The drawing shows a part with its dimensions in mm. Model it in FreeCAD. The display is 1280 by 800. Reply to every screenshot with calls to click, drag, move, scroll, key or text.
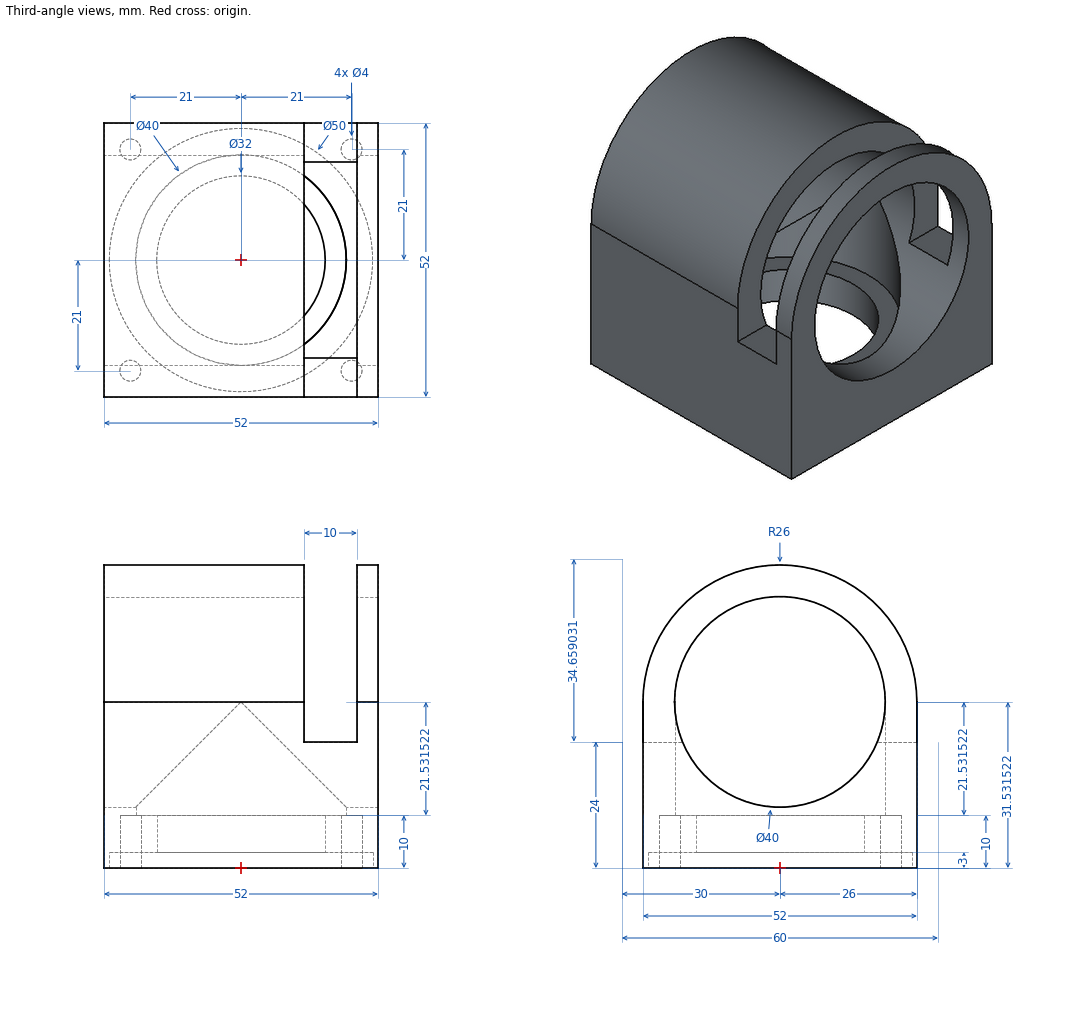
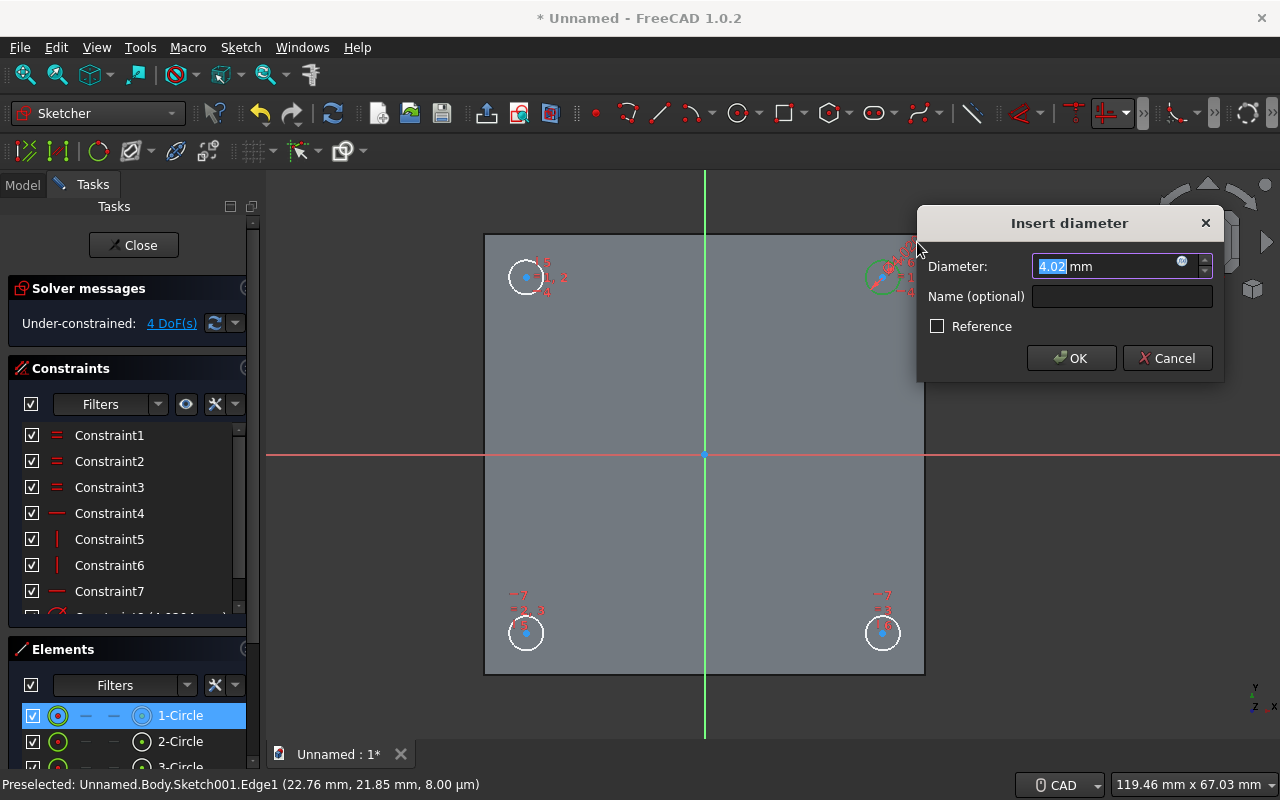
text(4)
key(Return)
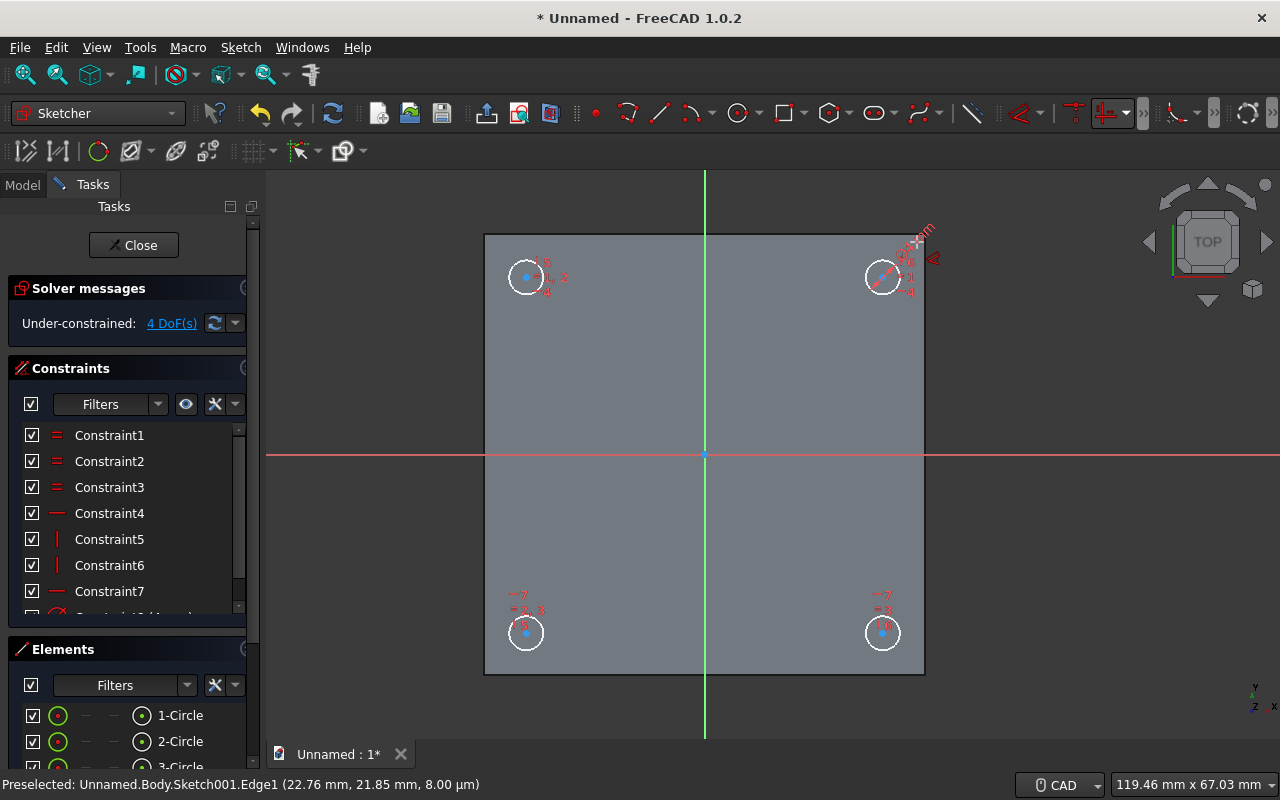
click(883, 277)
click(794, 243)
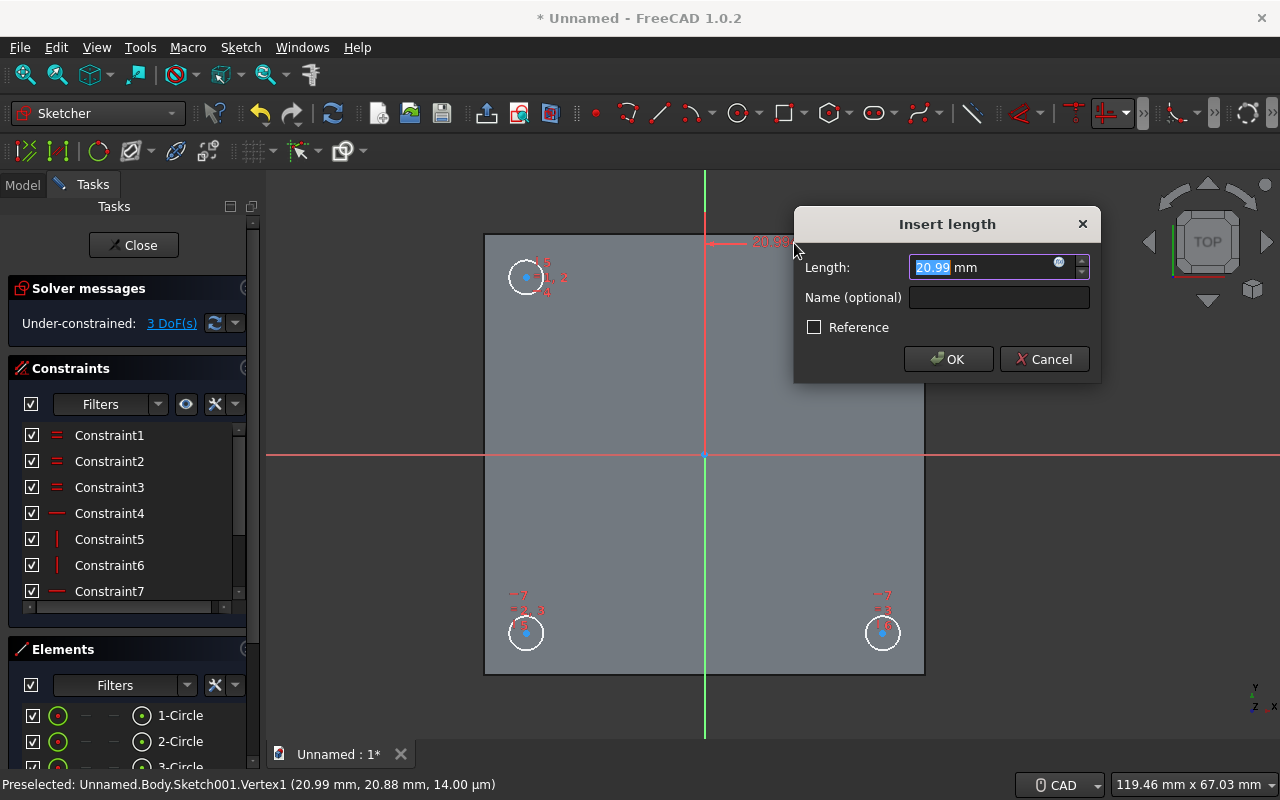
text(21)
key(Return)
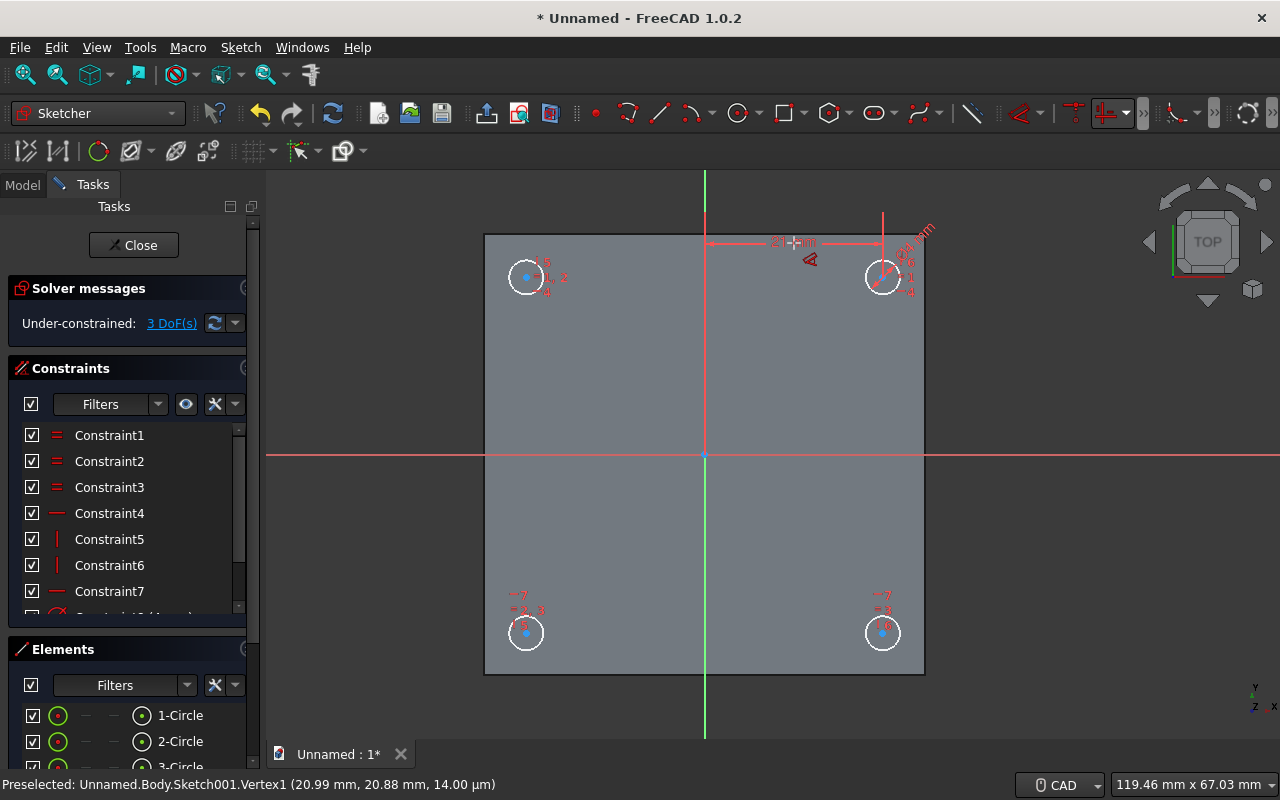
click(883, 277)
click(917, 366)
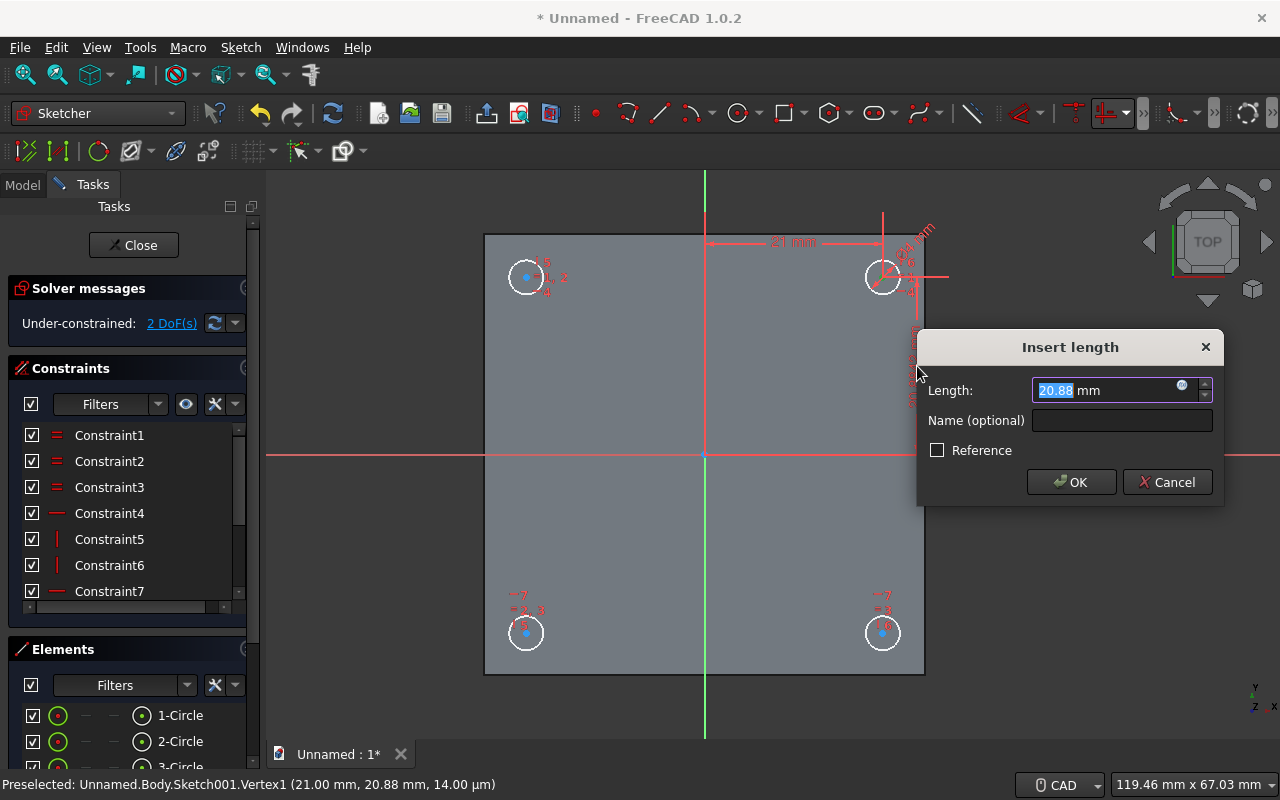
text(21)
key(Return)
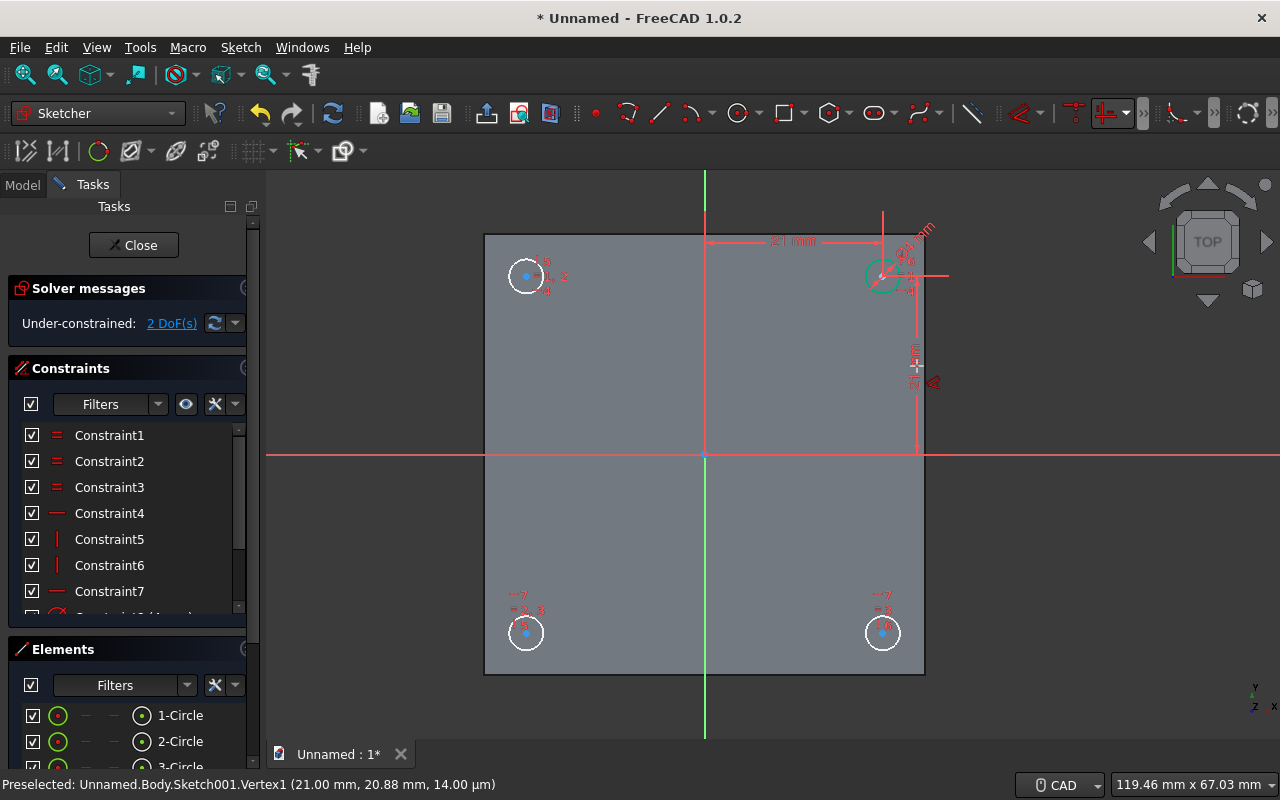
click(526, 276)
click(615, 242)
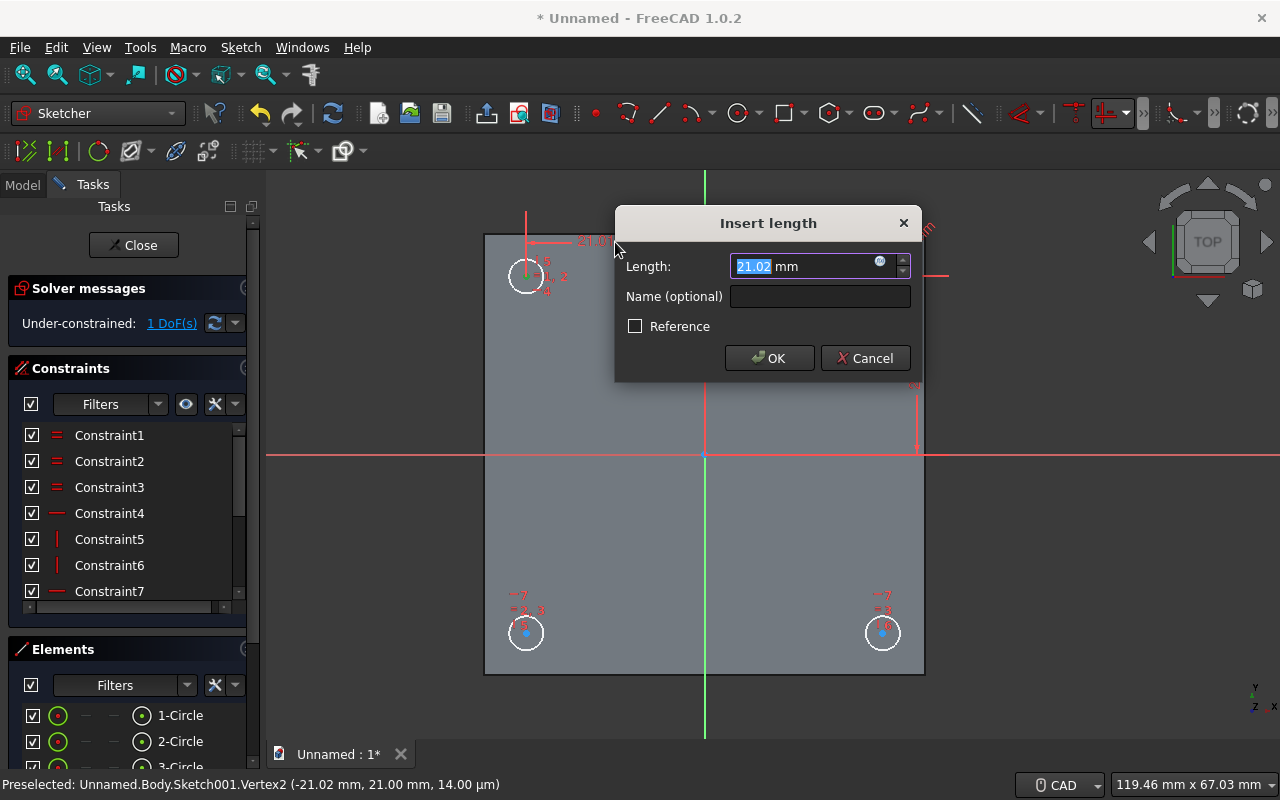
text(21)
key(Return)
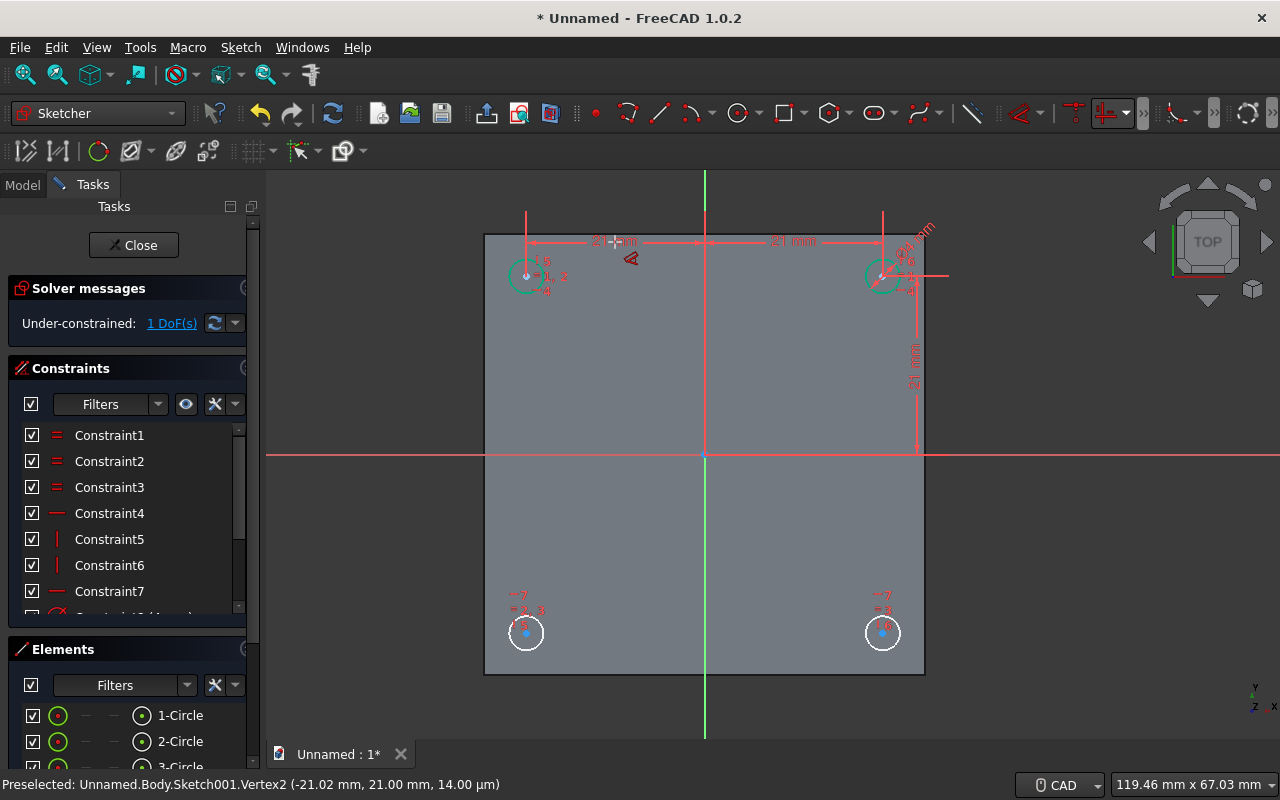
click(526, 633)
click(492, 544)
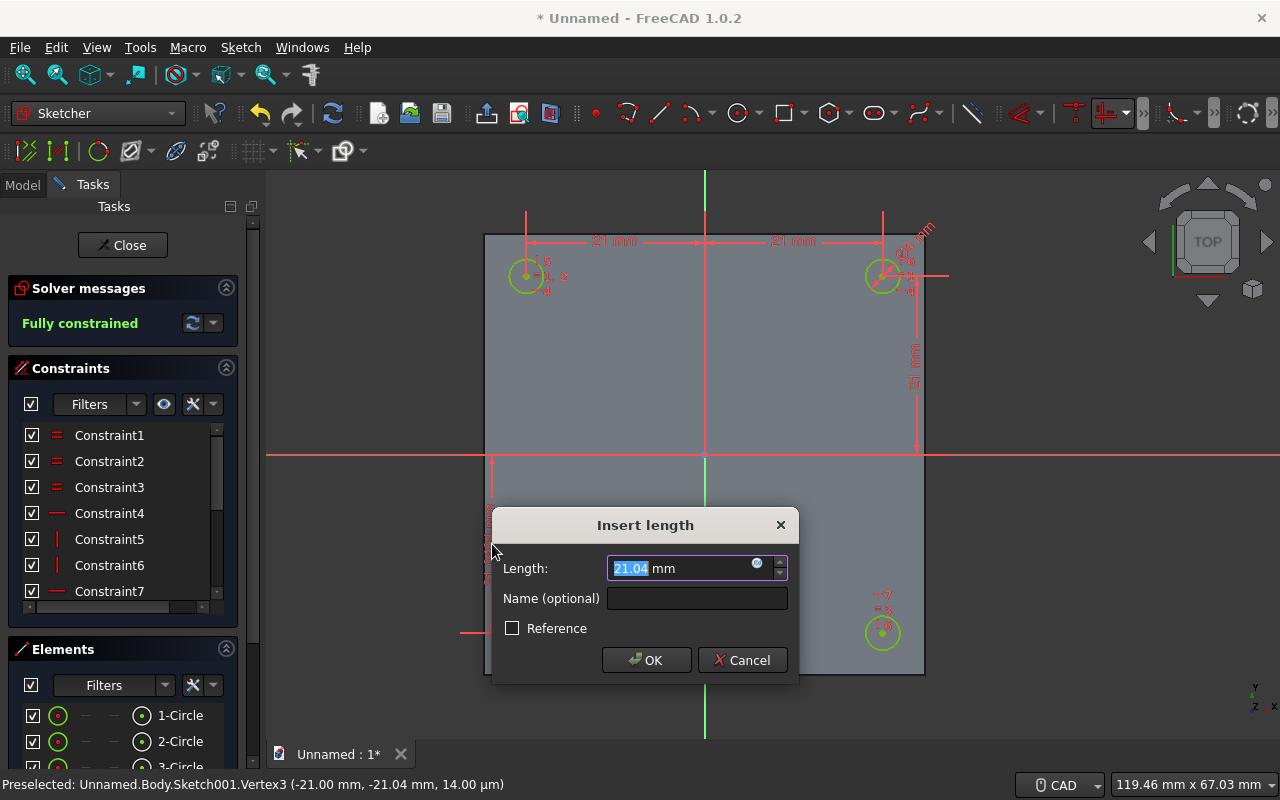
text(21)
key(Return)
key(Escape)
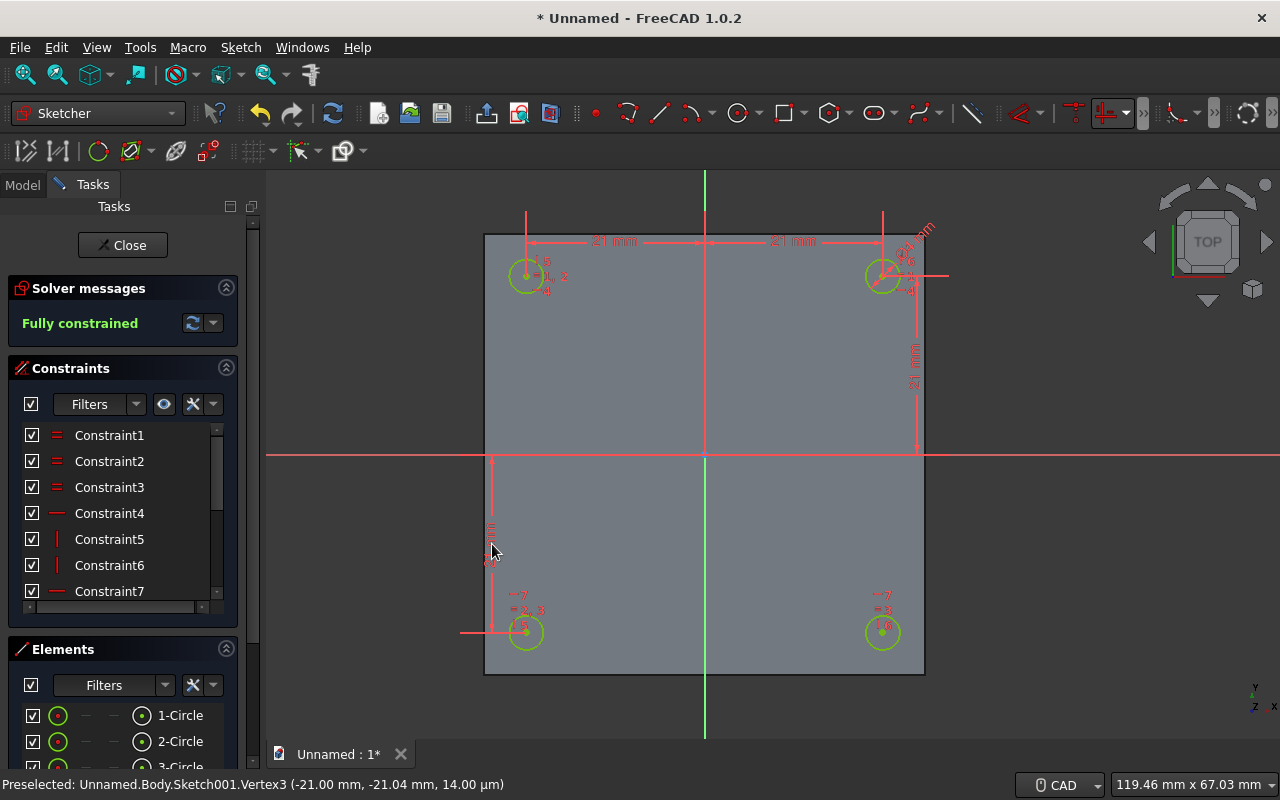
click(123, 245)